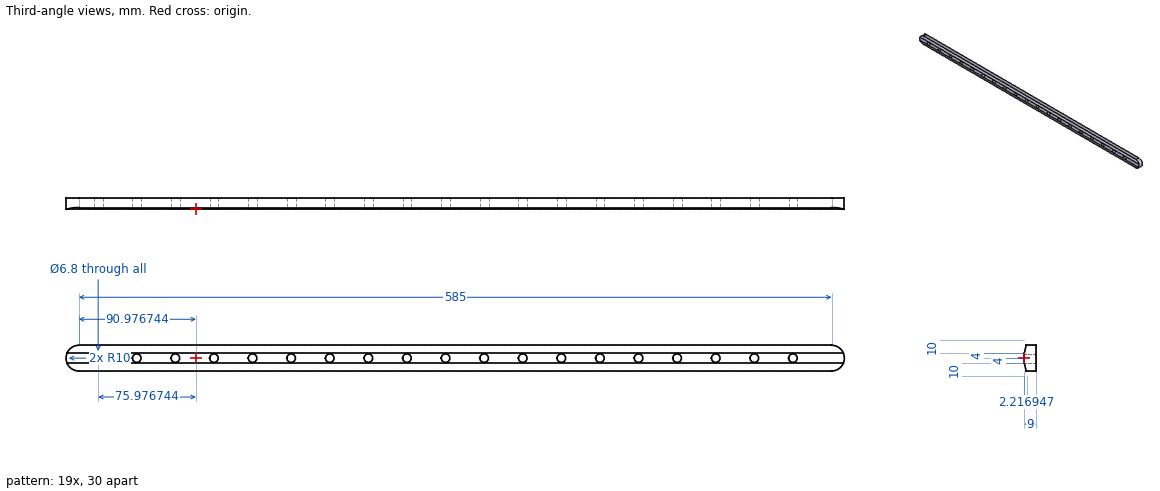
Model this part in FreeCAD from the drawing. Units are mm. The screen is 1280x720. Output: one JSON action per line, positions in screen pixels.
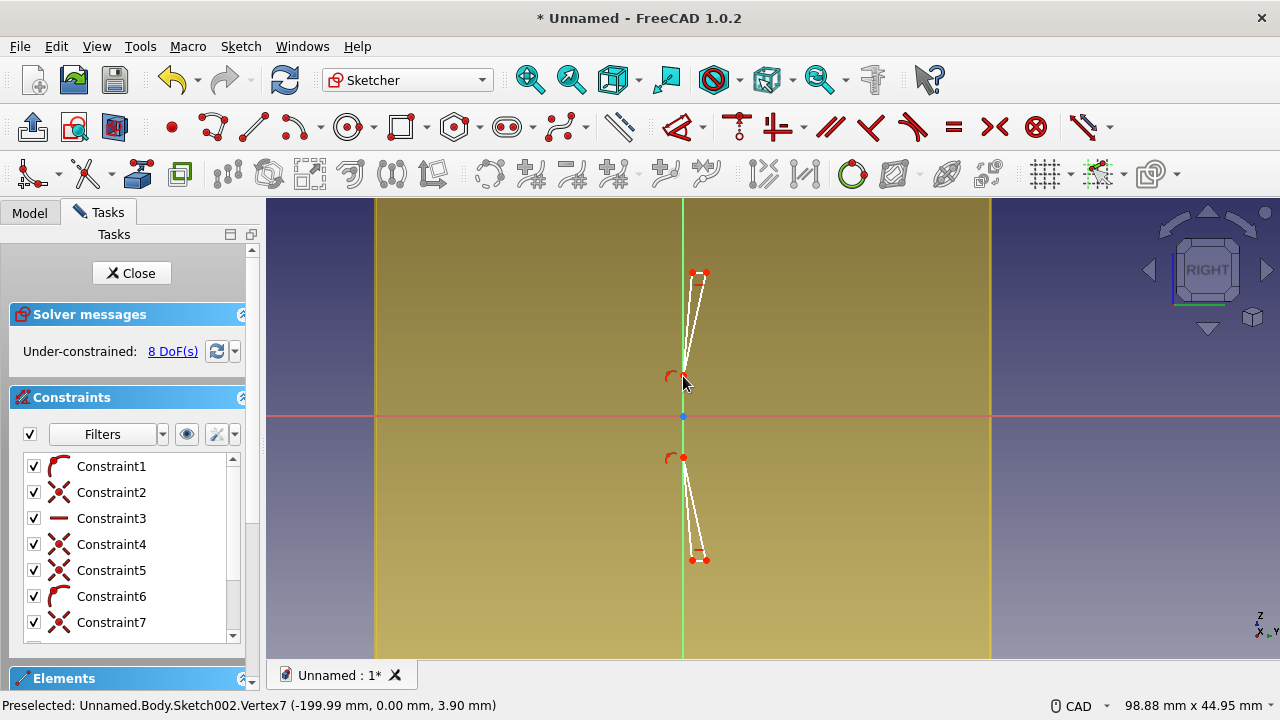
{"action": "scroll", "coordinate": [690, 540], "scroll_direction": "up", "scroll_amount": 4}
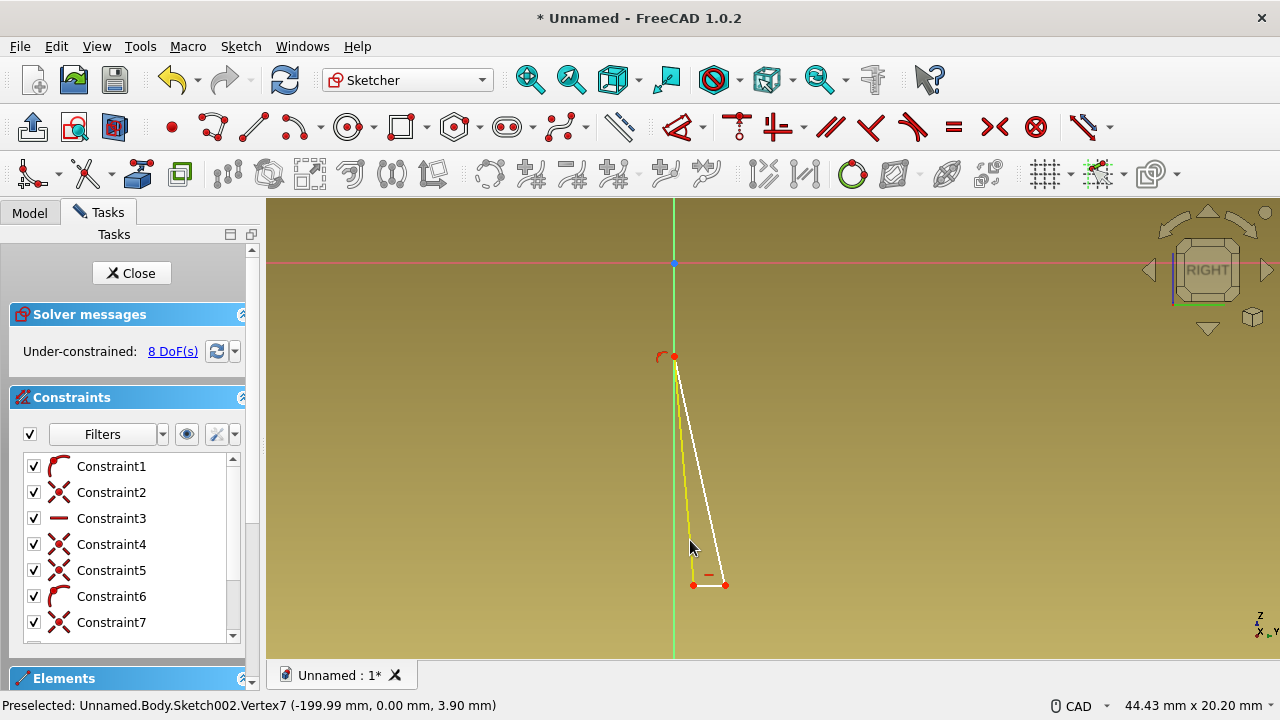
{"action": "left_click", "coordinate": [690, 540]}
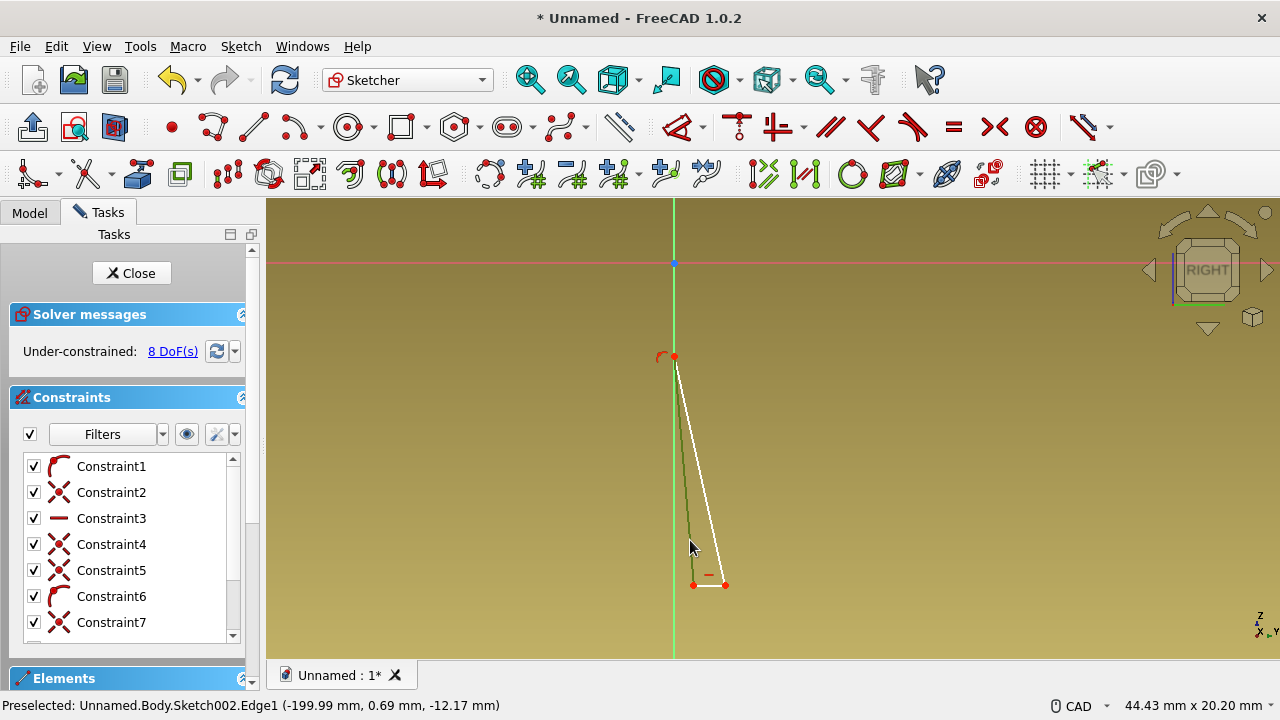
{"action": "left_click", "coordinate": [804, 128]}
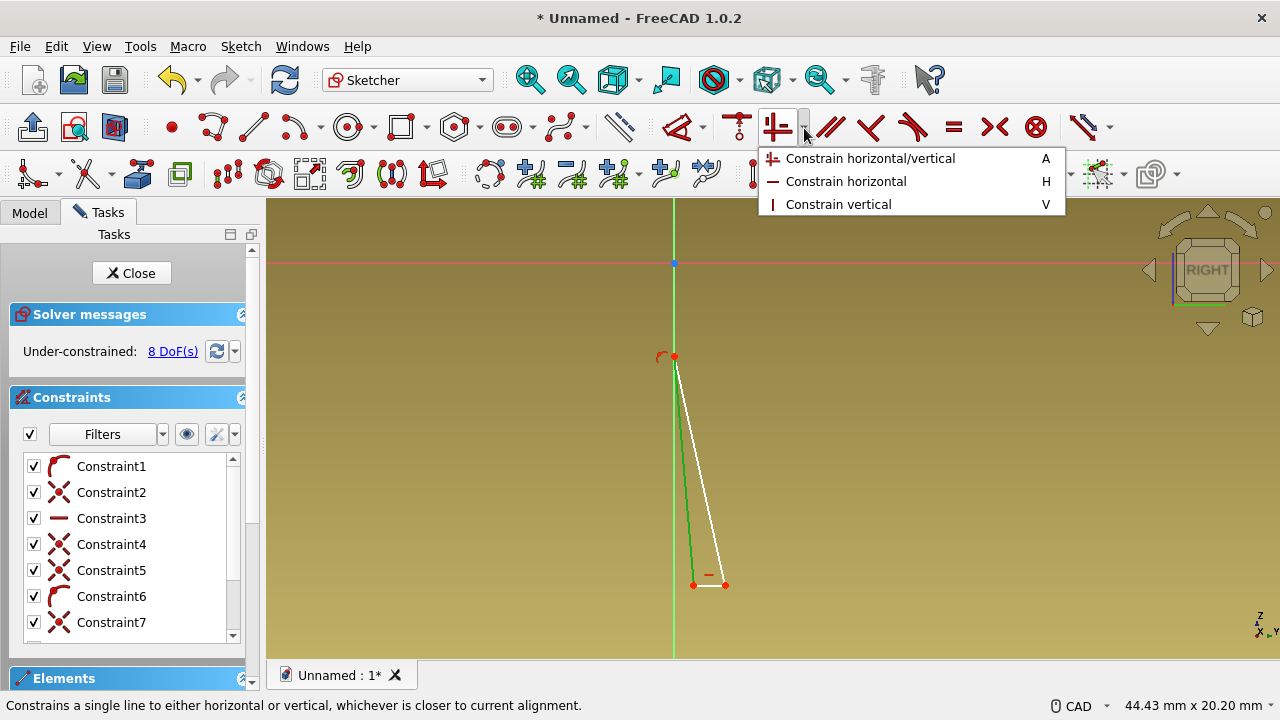
{"action": "left_click", "coordinate": [912, 204]}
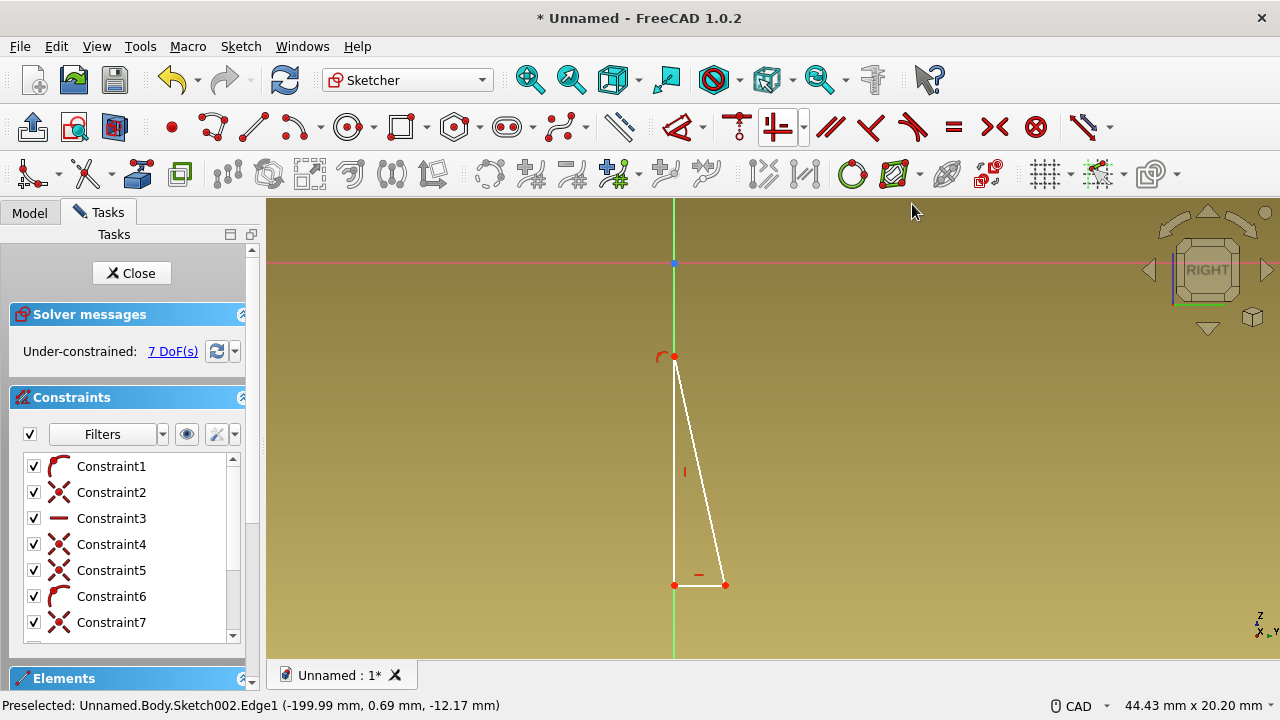
{"action": "scroll", "coordinate": [708, 563], "scroll_direction": "down", "scroll_amount": 4}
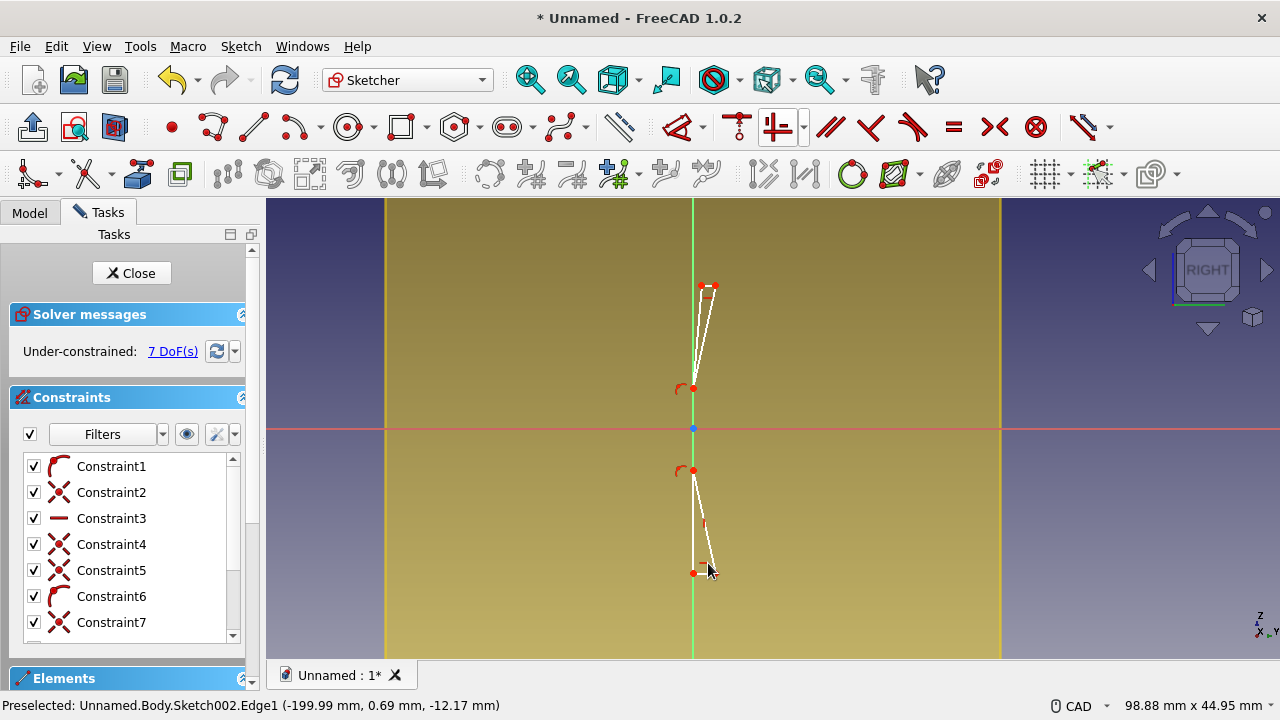
{"action": "scroll", "coordinate": [699, 317], "scroll_direction": "up", "scroll_amount": 5}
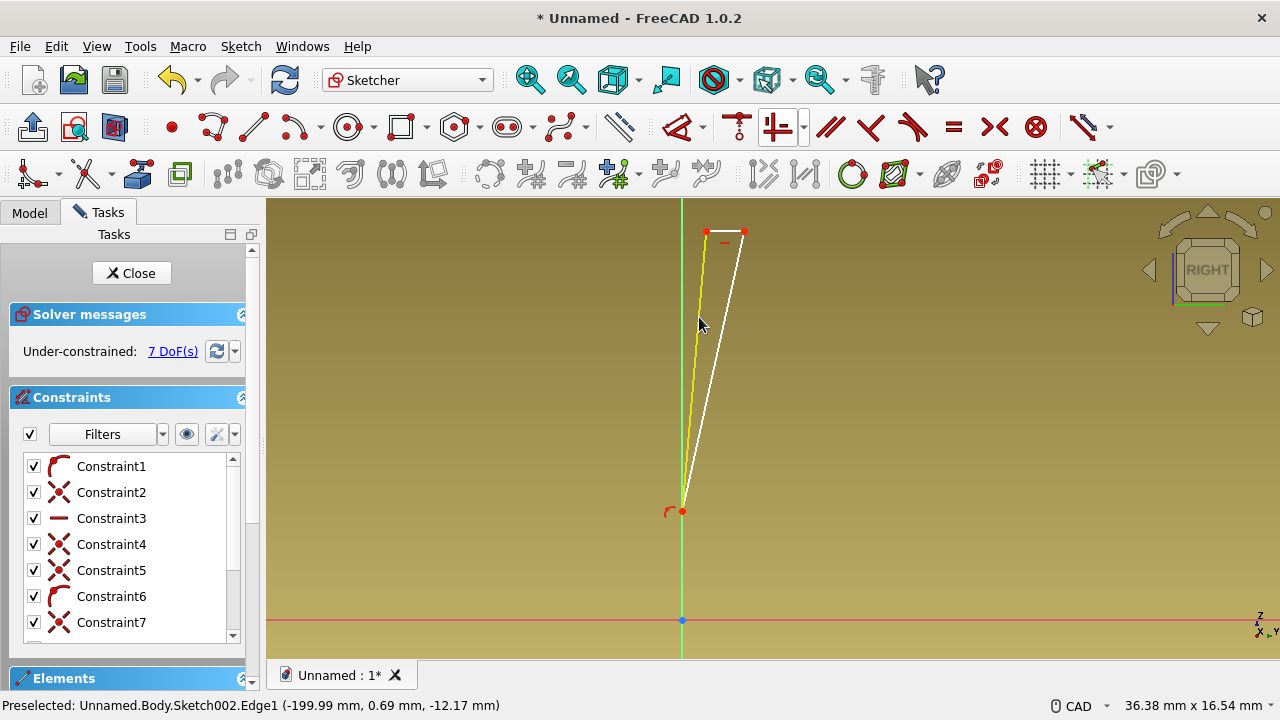
{"action": "left_click", "coordinate": [699, 315]}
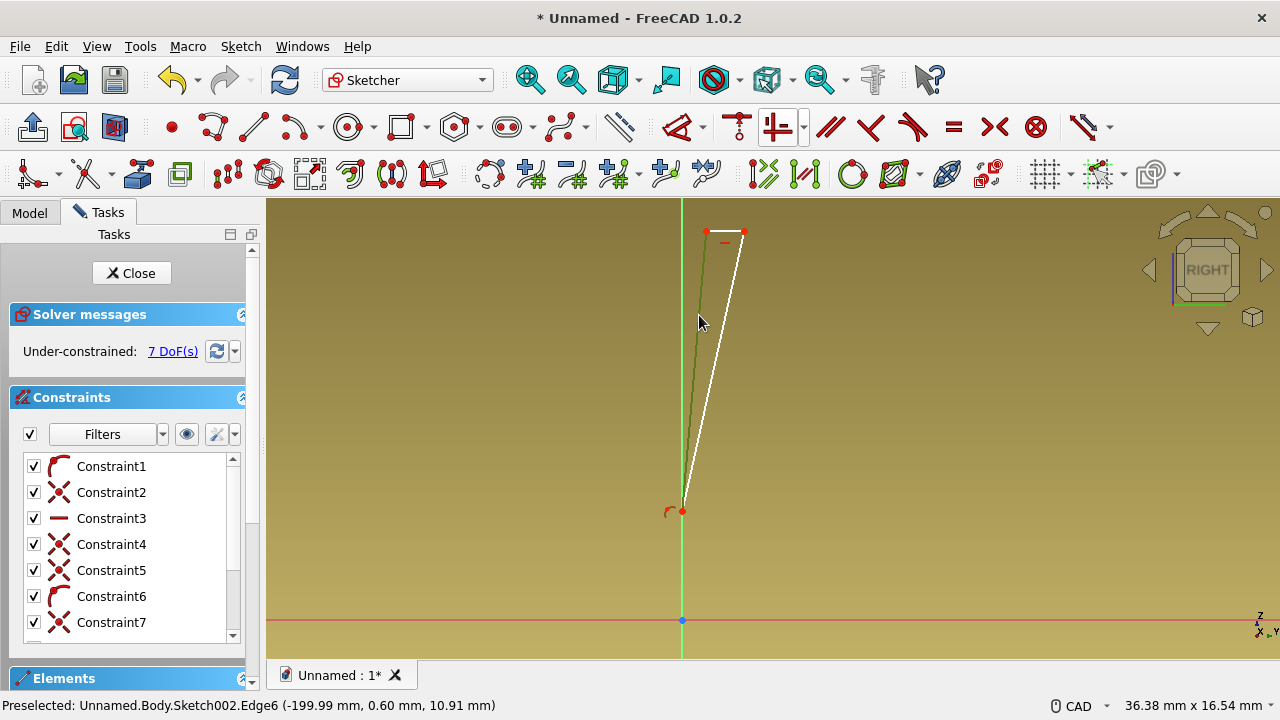
{"action": "key", "text": "v"}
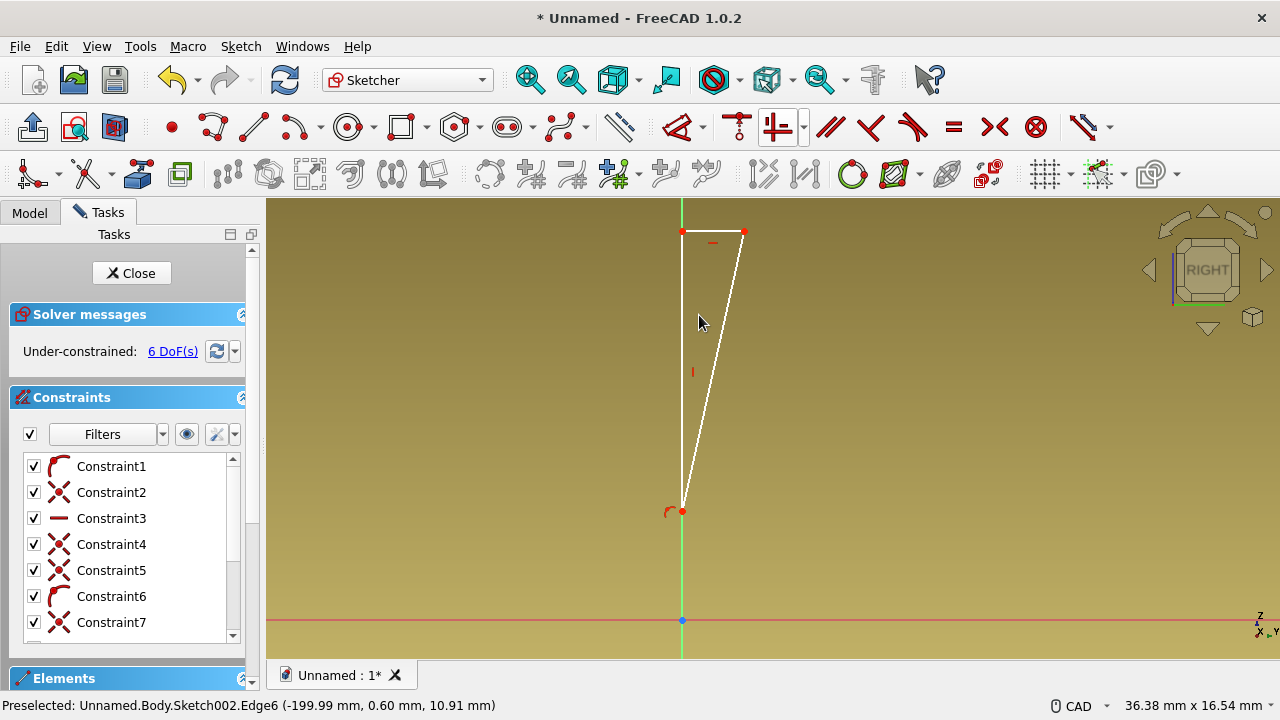
{"action": "left_click", "coordinate": [676, 128]}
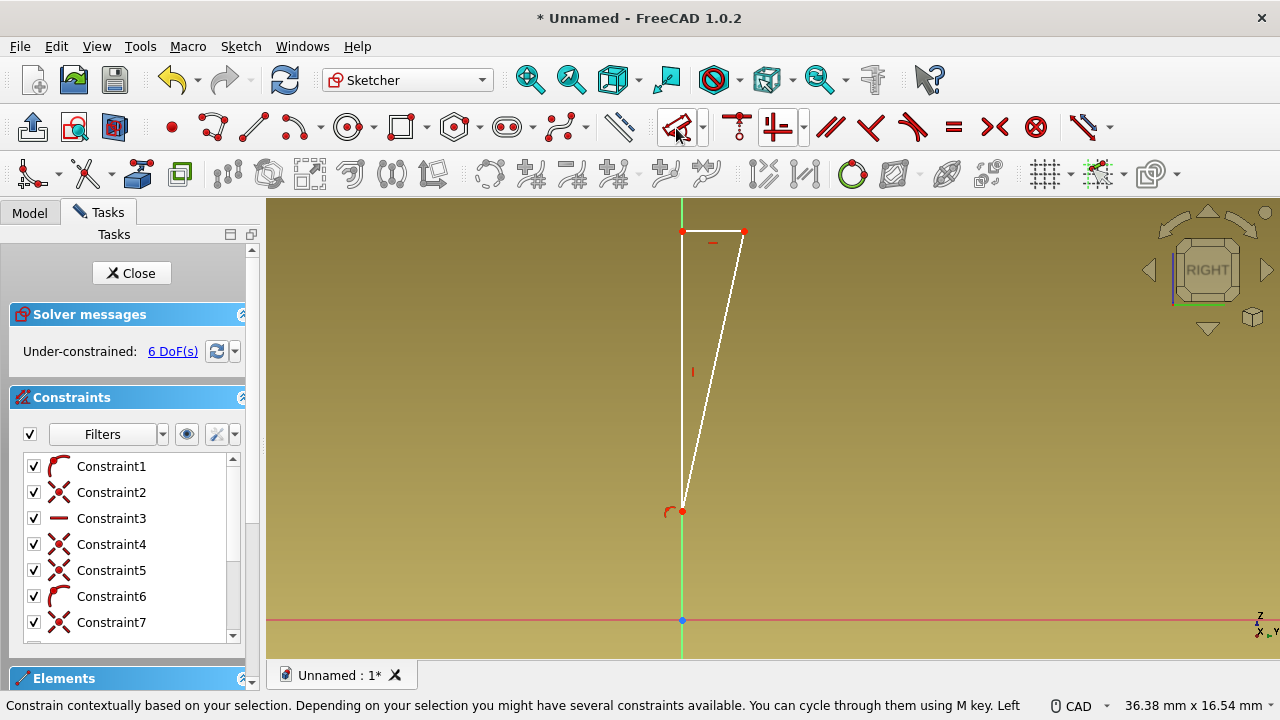
{"action": "scroll", "coordinate": [699, 317], "scroll_direction": "down", "scroll_amount": 5}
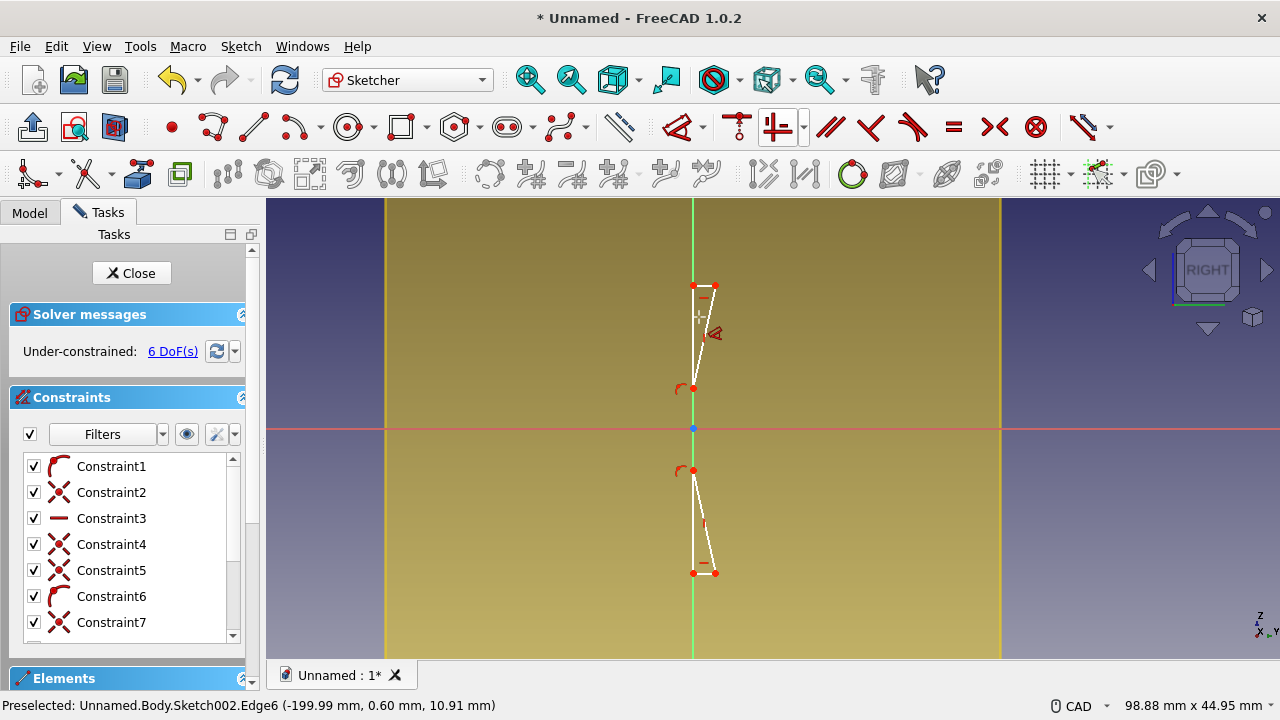
{"action": "scroll", "coordinate": [693, 502], "scroll_direction": "up", "scroll_amount": 4}